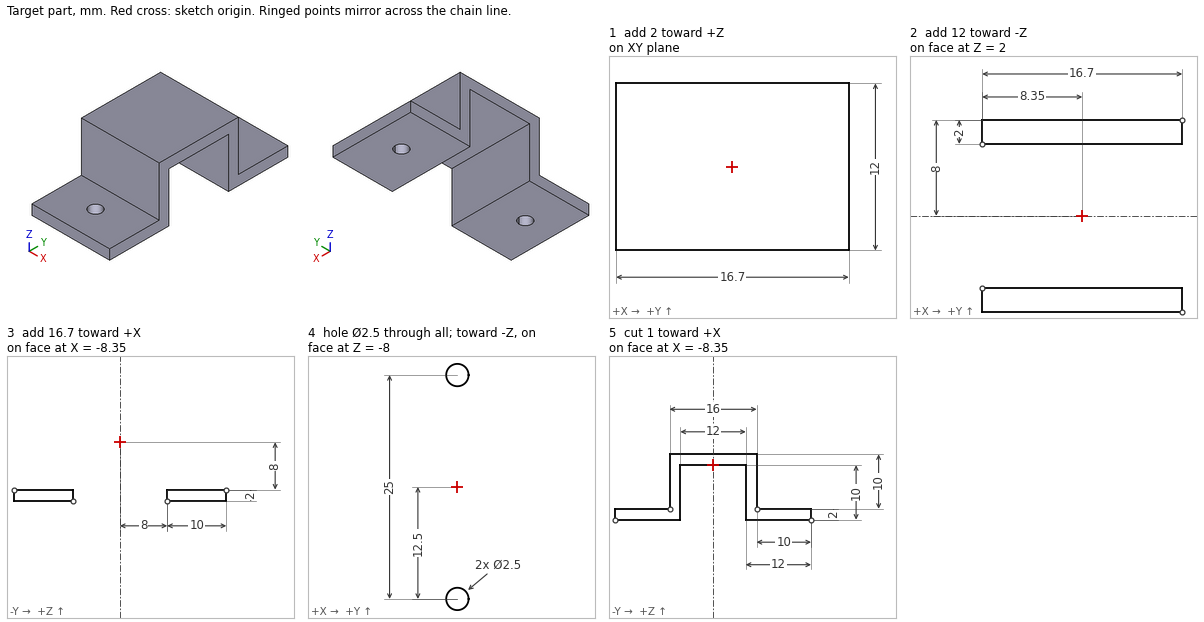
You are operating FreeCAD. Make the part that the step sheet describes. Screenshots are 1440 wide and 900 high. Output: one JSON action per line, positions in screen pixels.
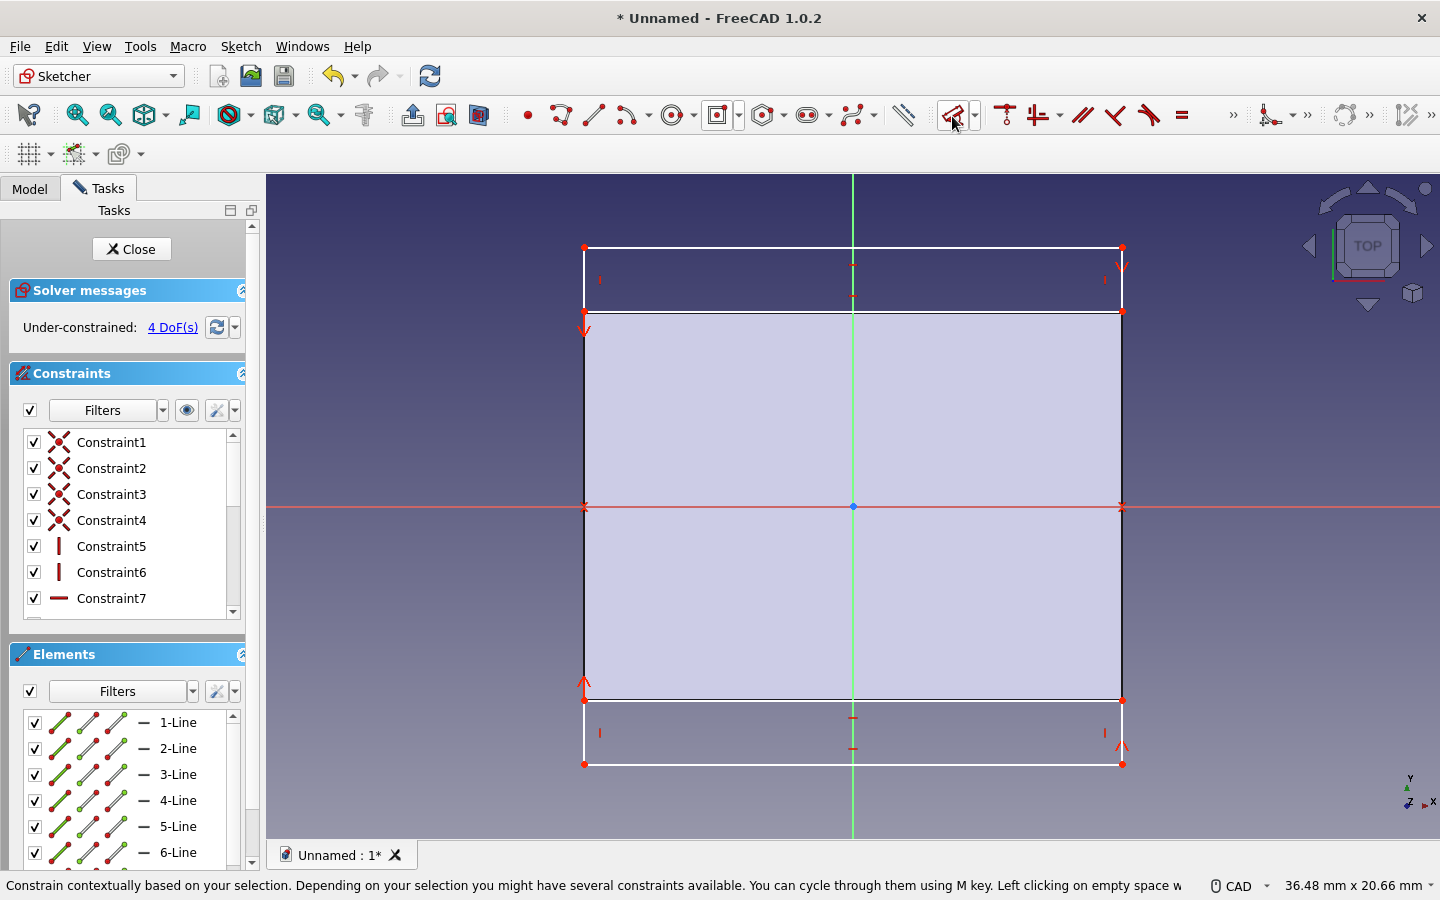
{"action": "left_click", "coordinate": [584, 267]}
{"action": "left_click", "coordinate": [550, 280]}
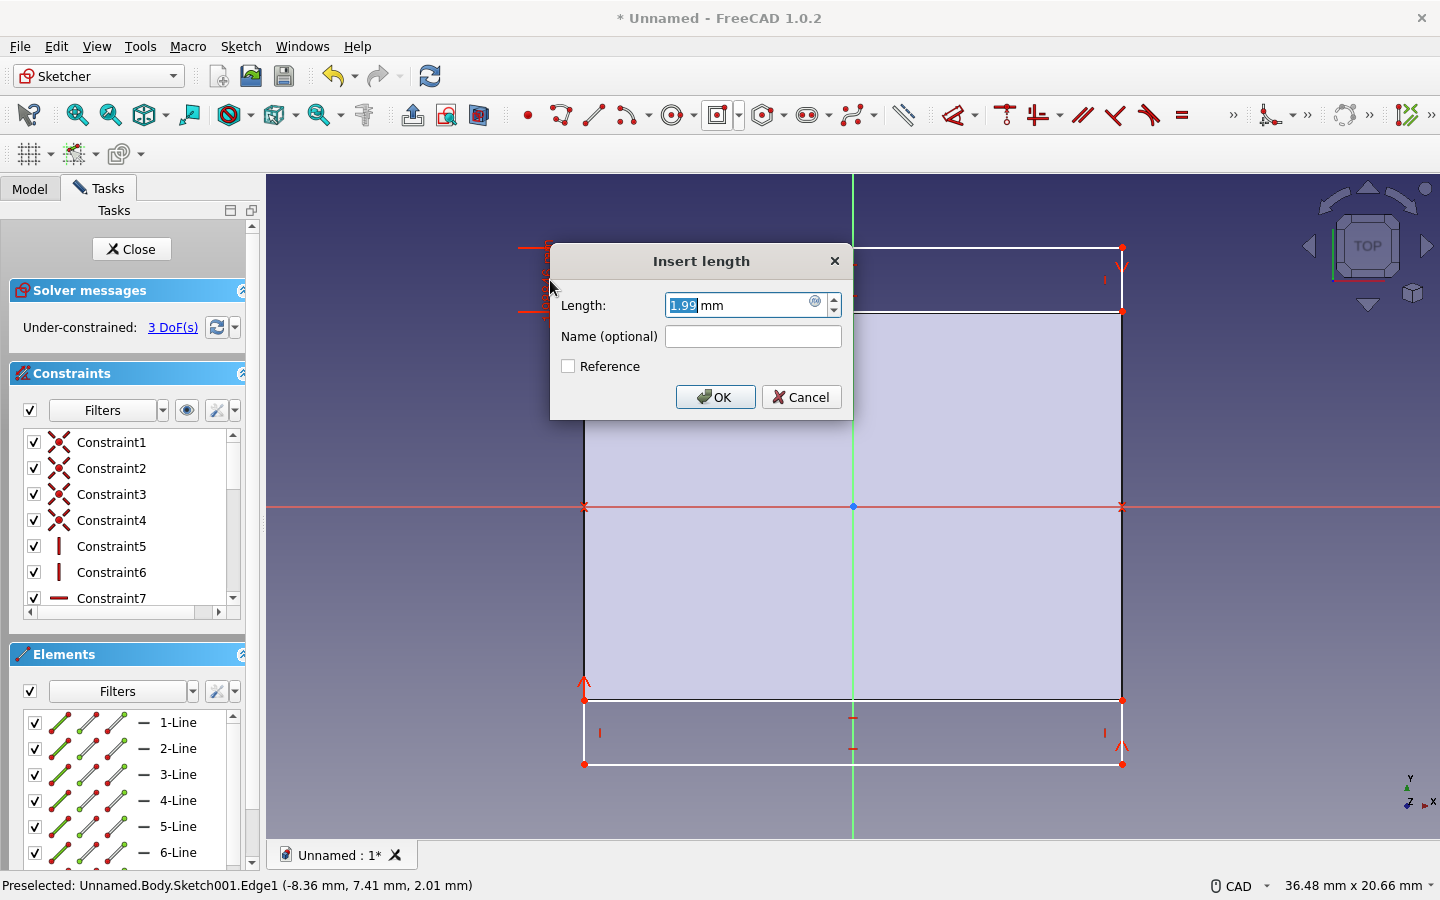
{"action": "type", "text": "2"}
{"action": "key", "text": "Return"}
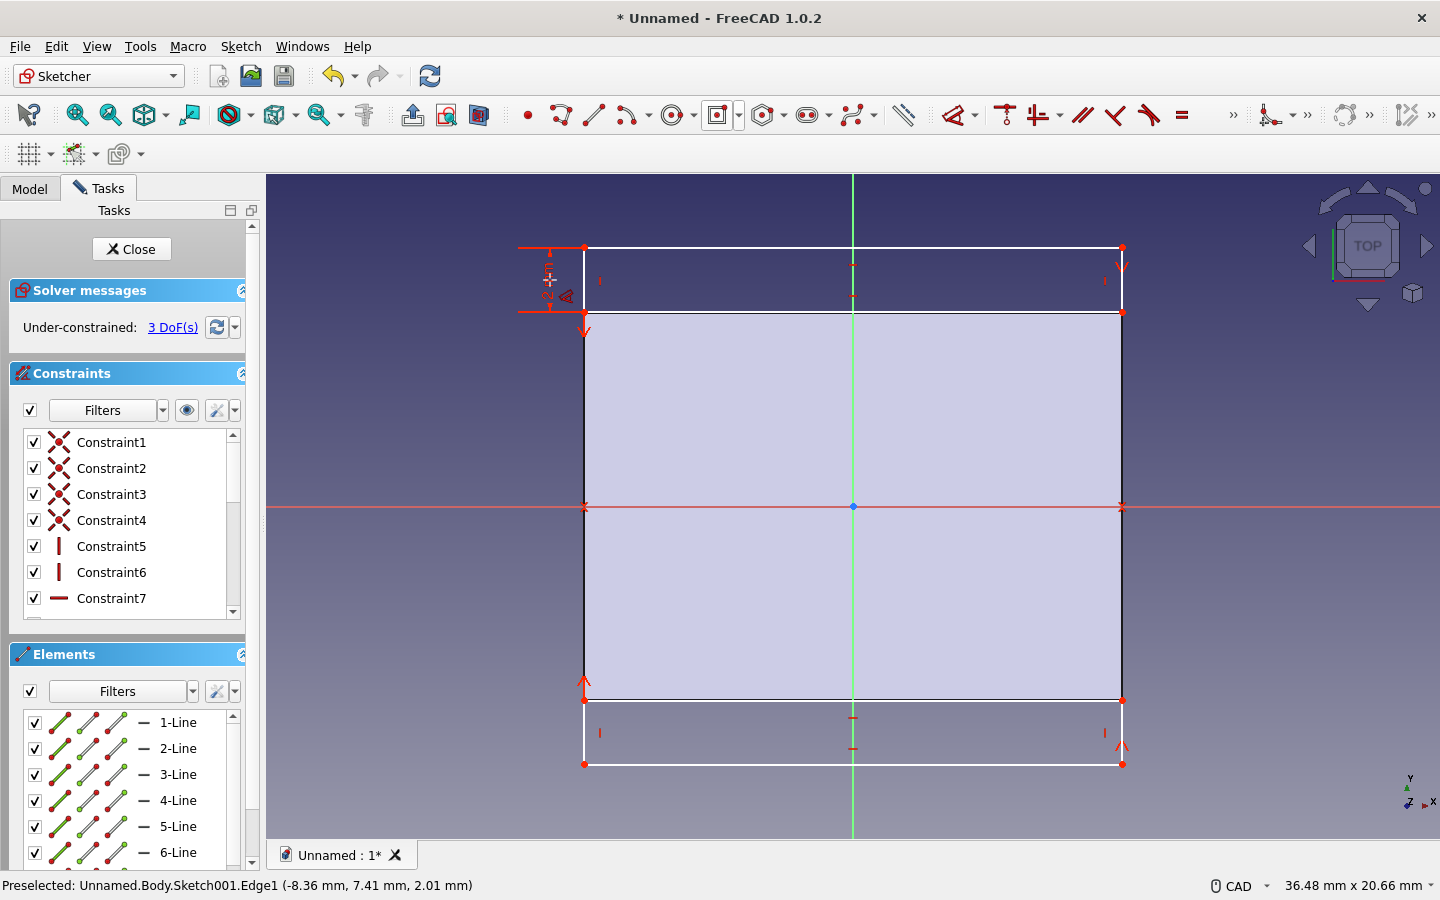
{"action": "left_click", "coordinate": [584, 248]}
{"action": "left_click", "coordinate": [550, 377]}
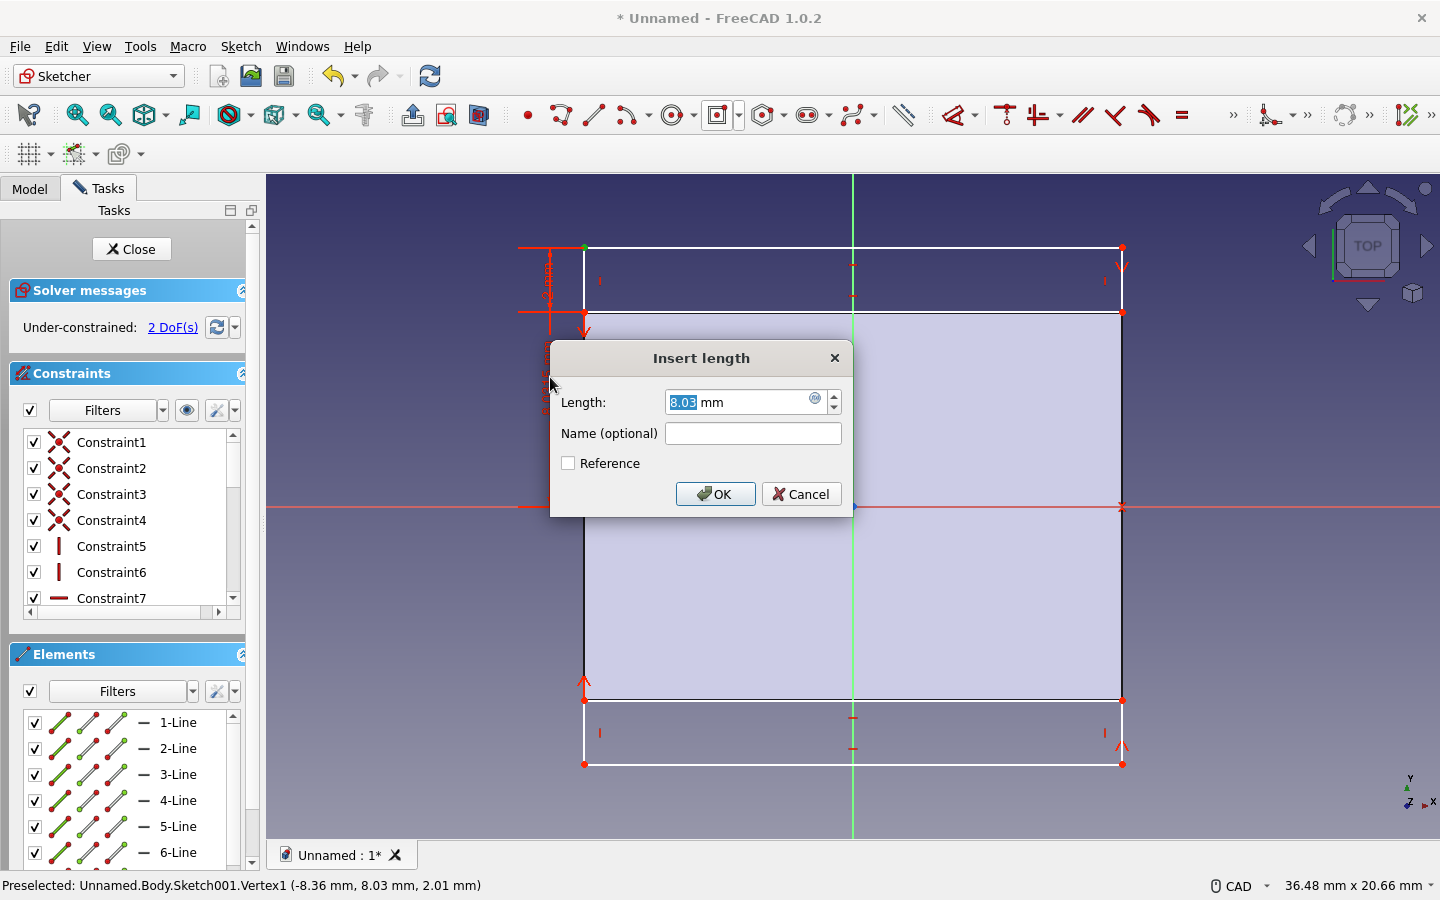
{"action": "type", "text": "8"}
{"action": "key", "text": "Return"}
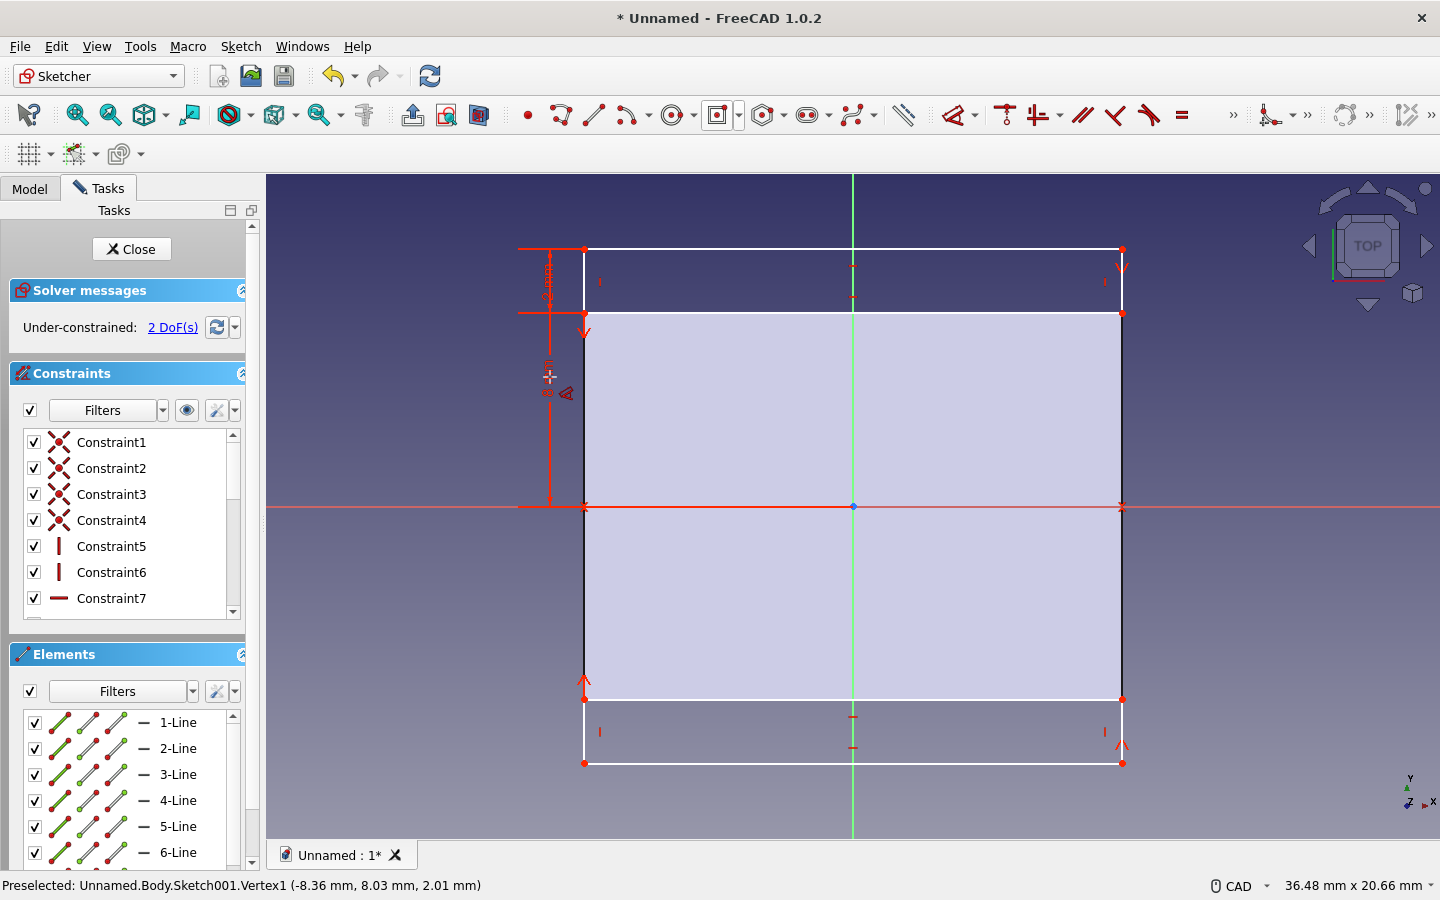
{"action": "left_click", "coordinate": [745, 313]}
{"action": "left_click", "coordinate": [729, 279]}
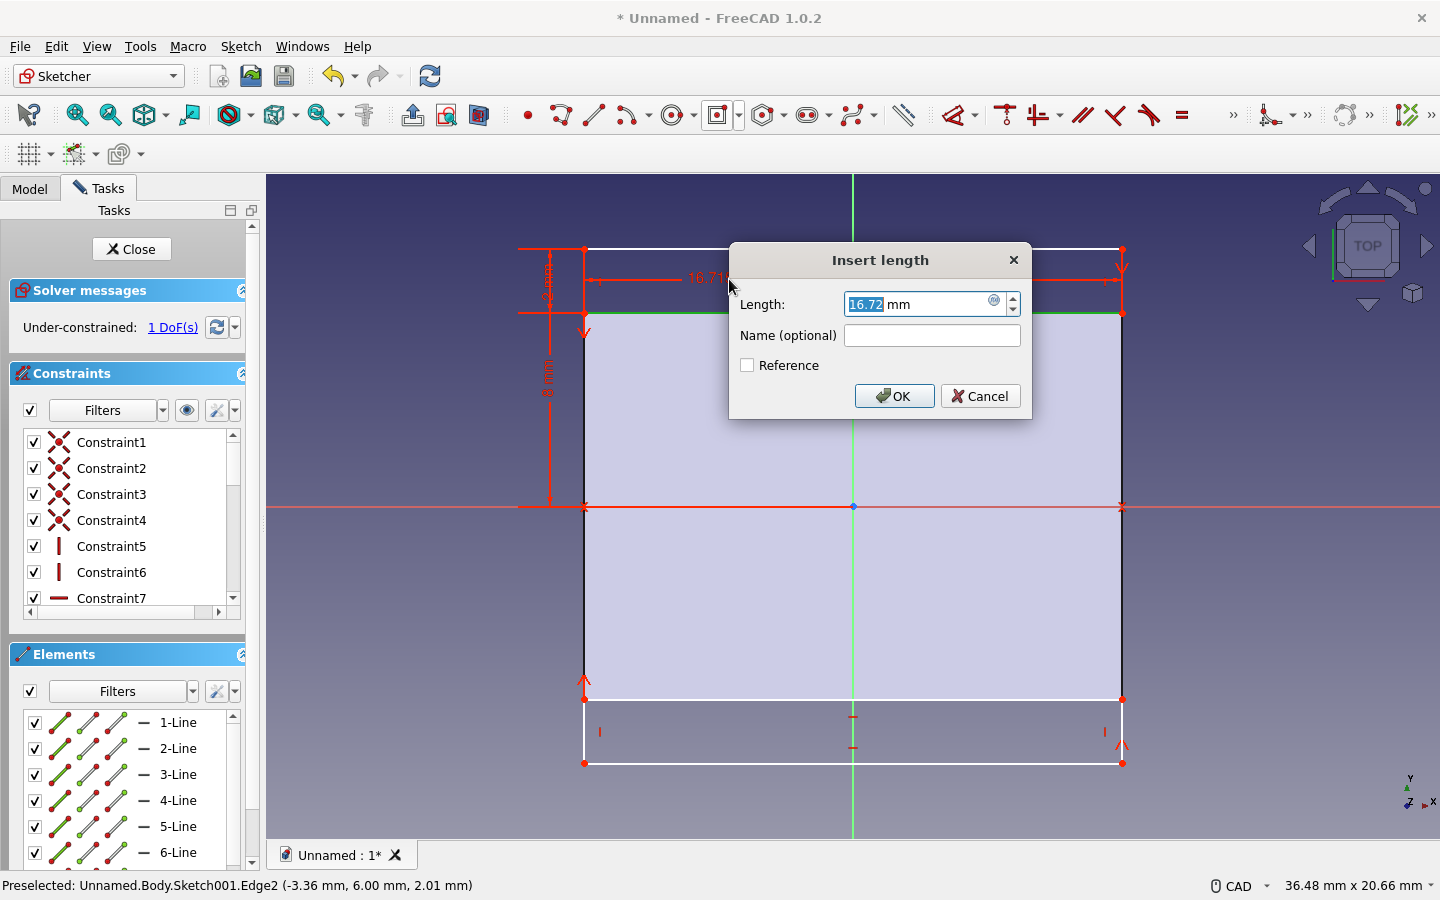
{"action": "type", "text": "16.7"}
{"action": "key", "text": "Return"}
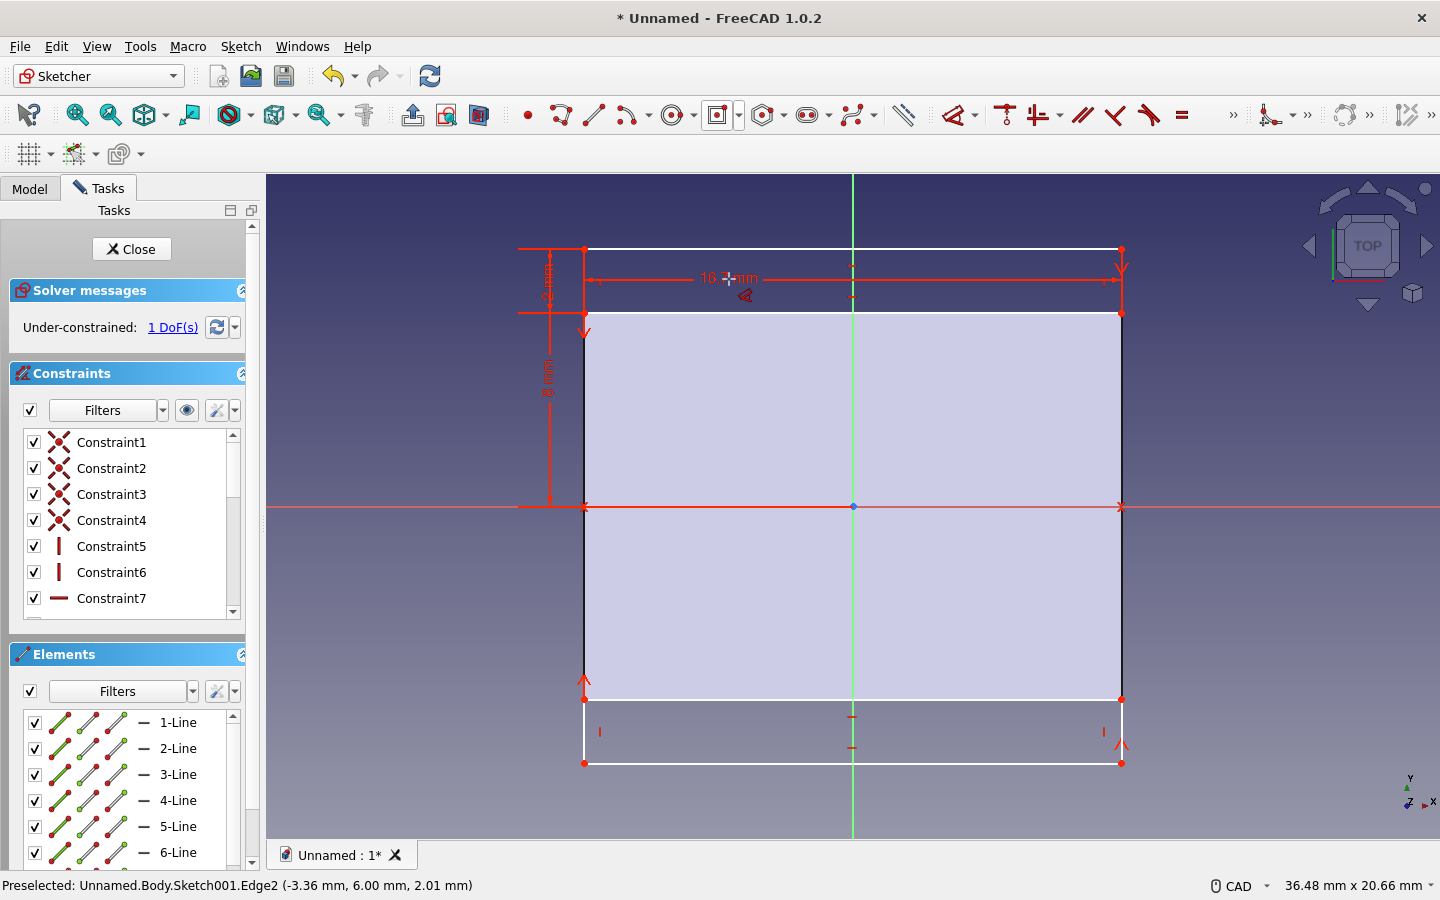
{"action": "left_click", "coordinate": [584, 249]}
{"action": "left_click", "coordinate": [719, 215]}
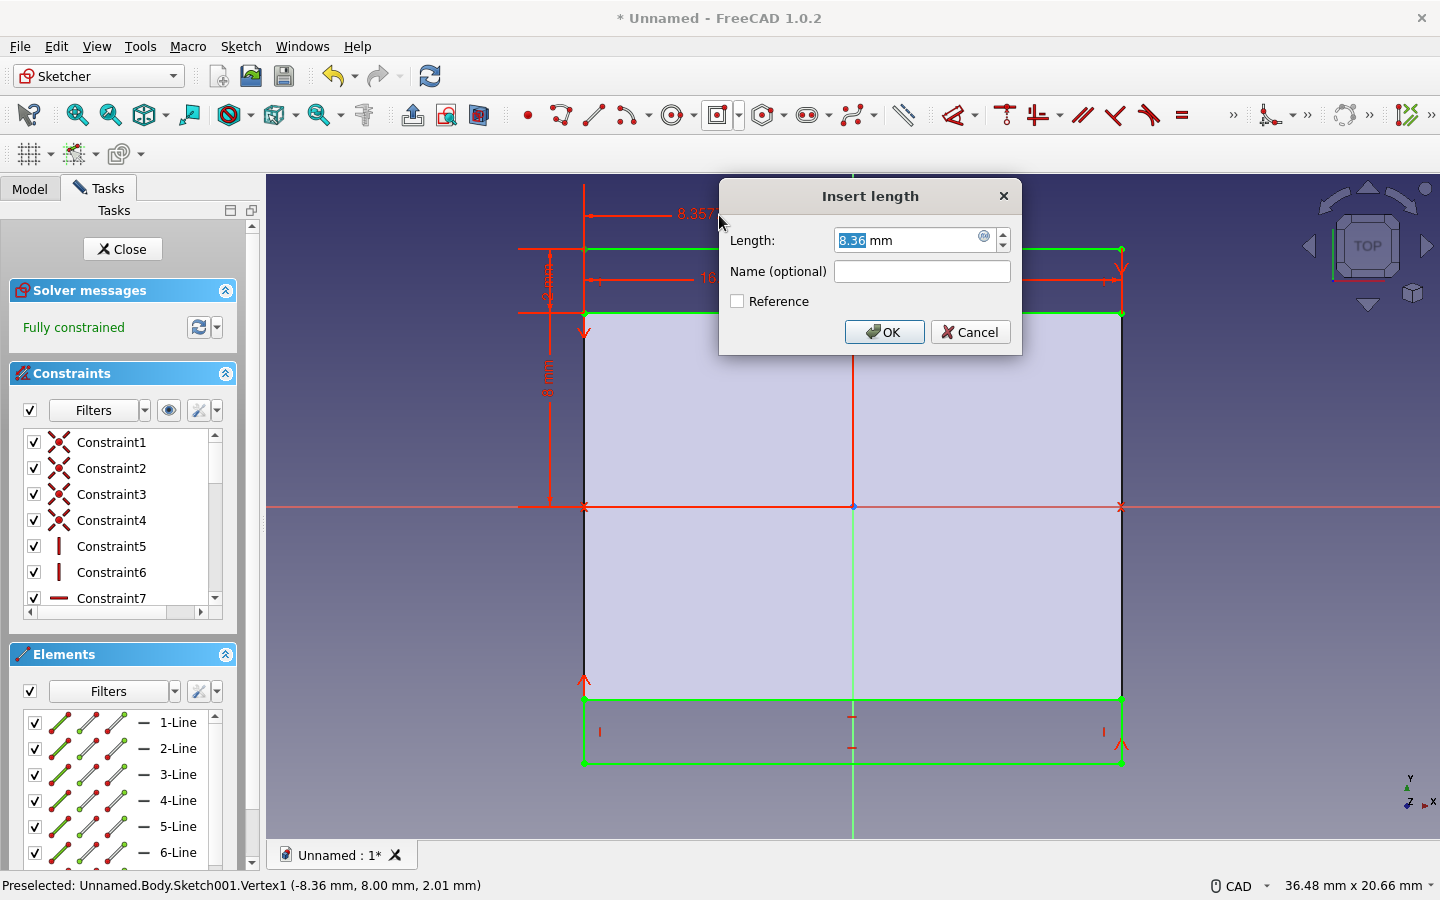
{"action": "type", "text": "8.35"}
{"action": "key", "text": "Return"}
{"action": "key", "text": "Escape"}